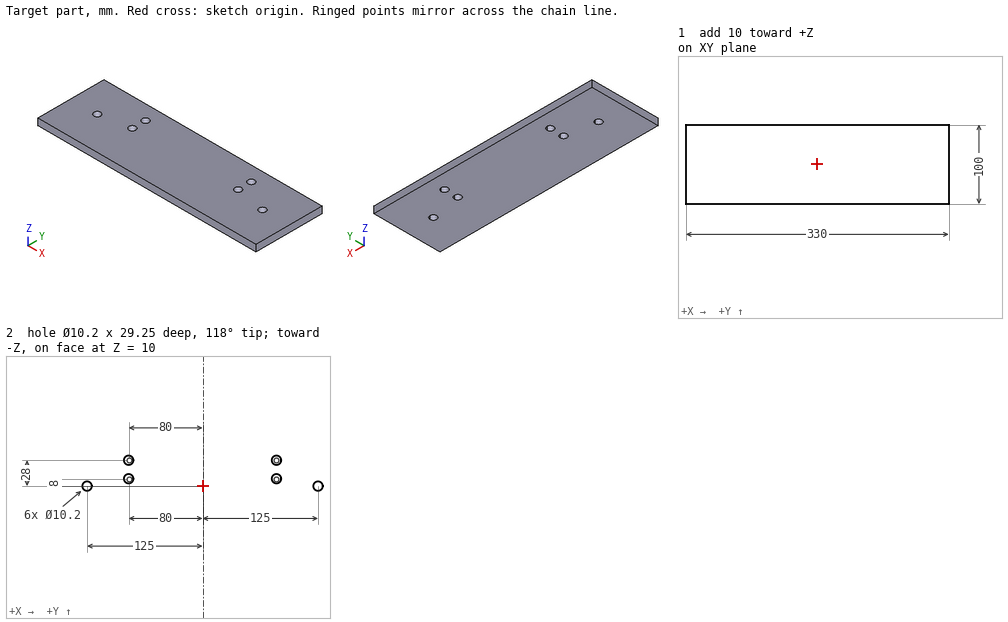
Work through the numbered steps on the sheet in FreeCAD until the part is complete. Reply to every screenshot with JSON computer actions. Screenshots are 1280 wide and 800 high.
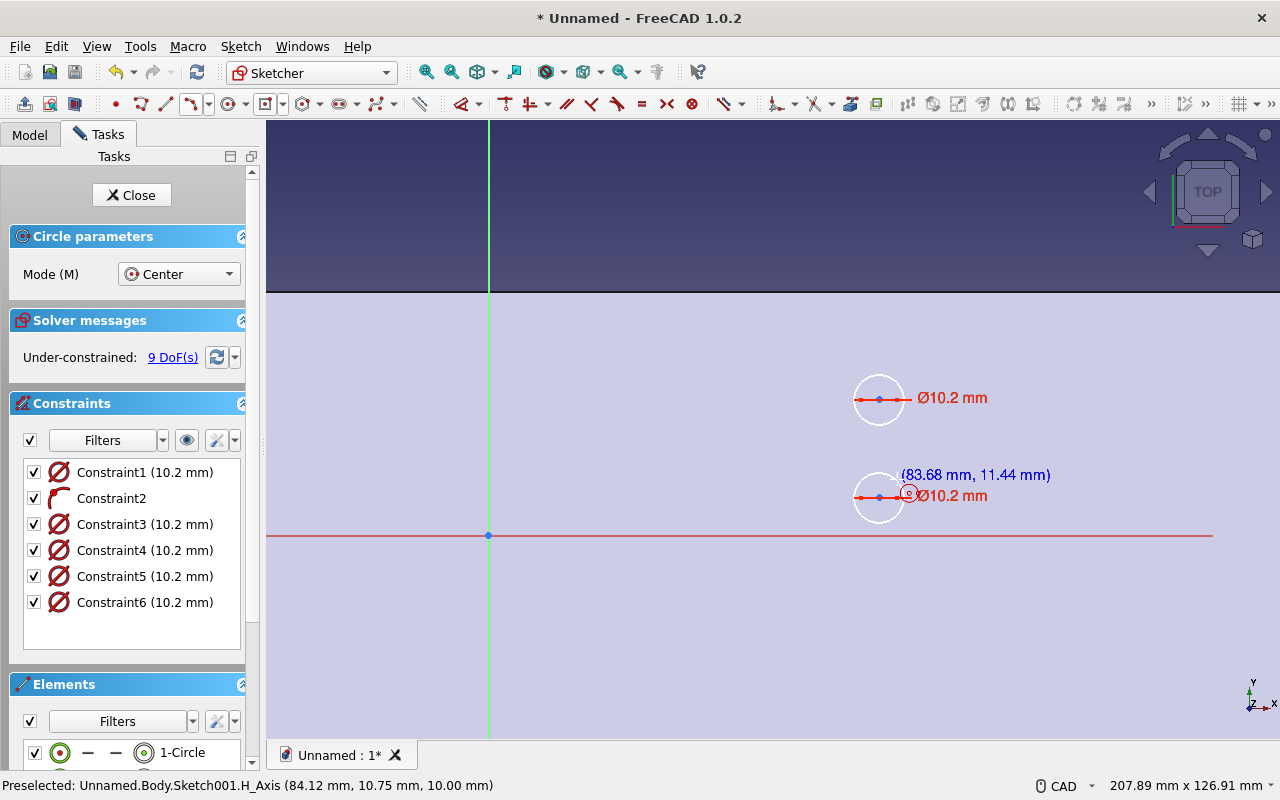
{"action": "left_click", "coordinate": [1099, 536]}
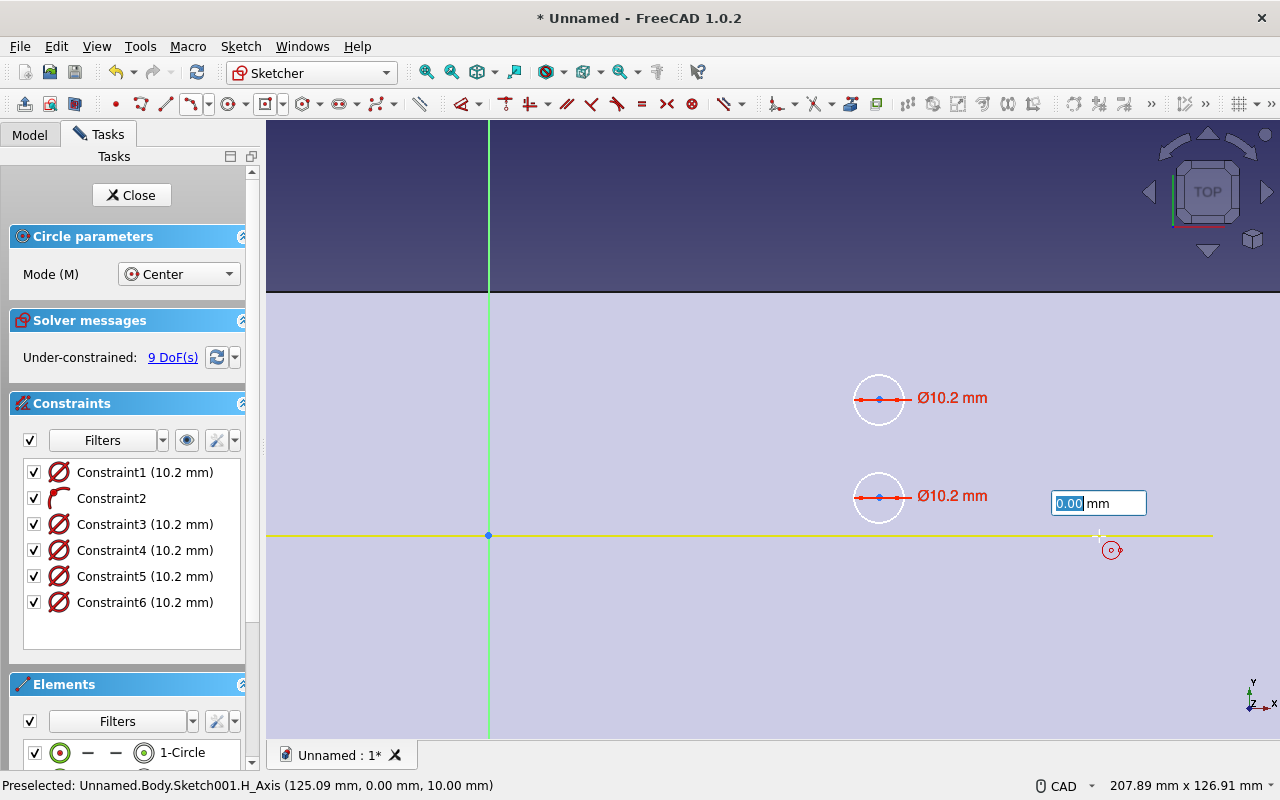
{"action": "scroll", "coordinate": [880, 398], "scroll_direction": "down", "scroll_amount": 4}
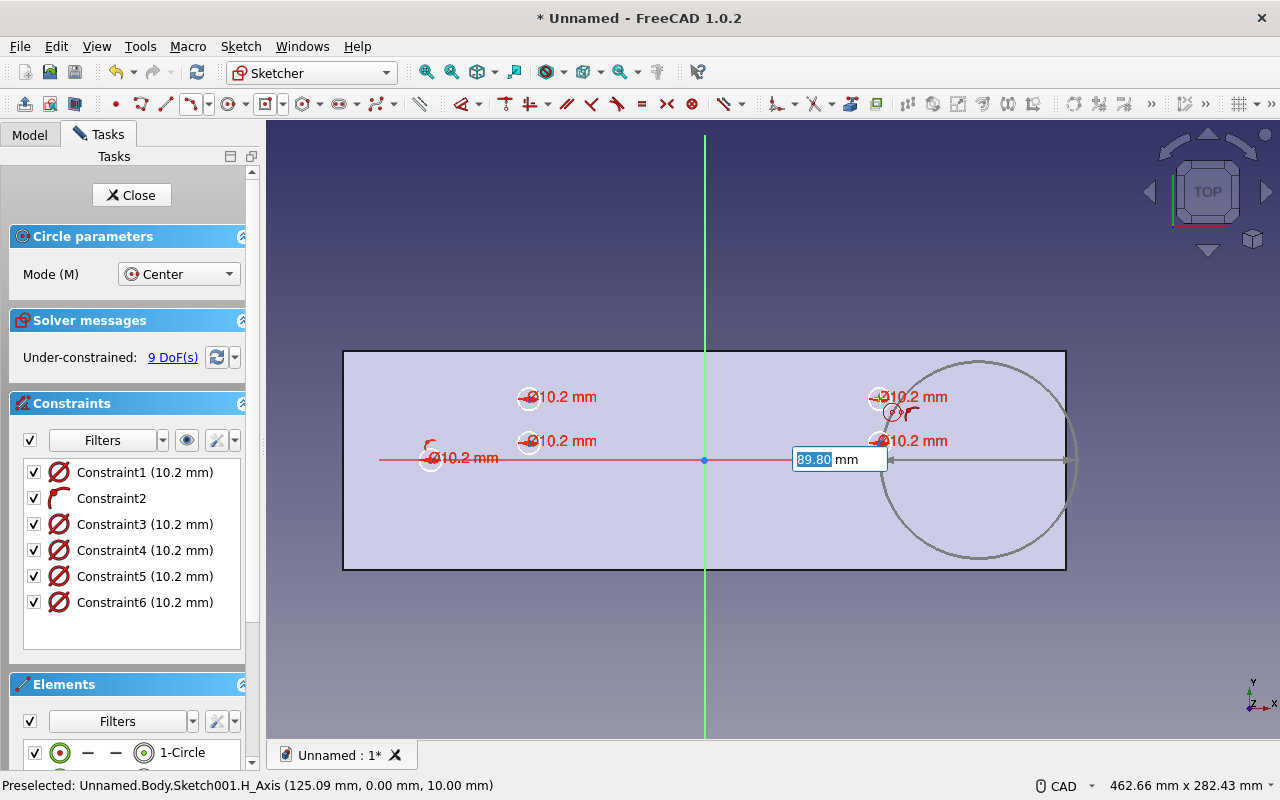
{"action": "scroll", "coordinate": [986, 452], "scroll_direction": "up", "scroll_amount": 4}
{"action": "mouse_move", "coordinate": [986, 452]}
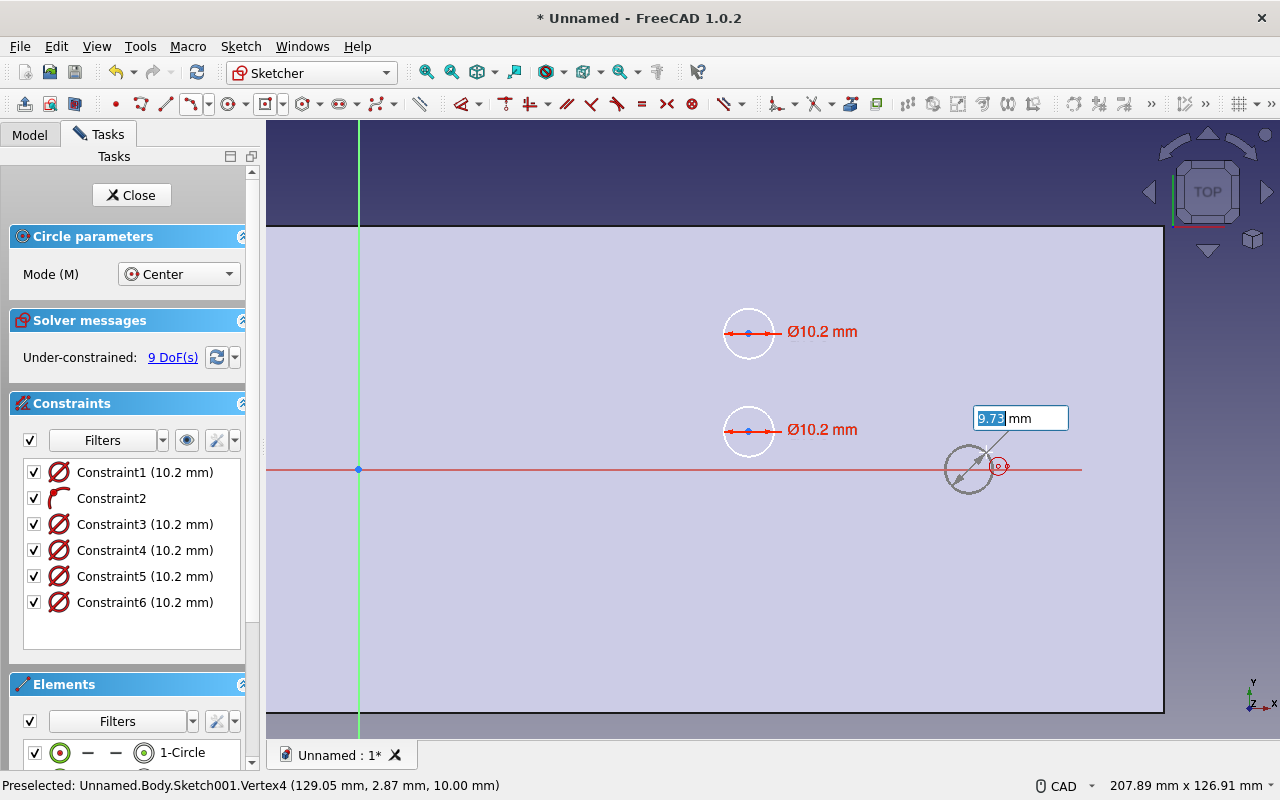
{"action": "type", "text": "10.2"}
{"action": "key", "text": "Return"}
{"action": "key", "text": "Escape"}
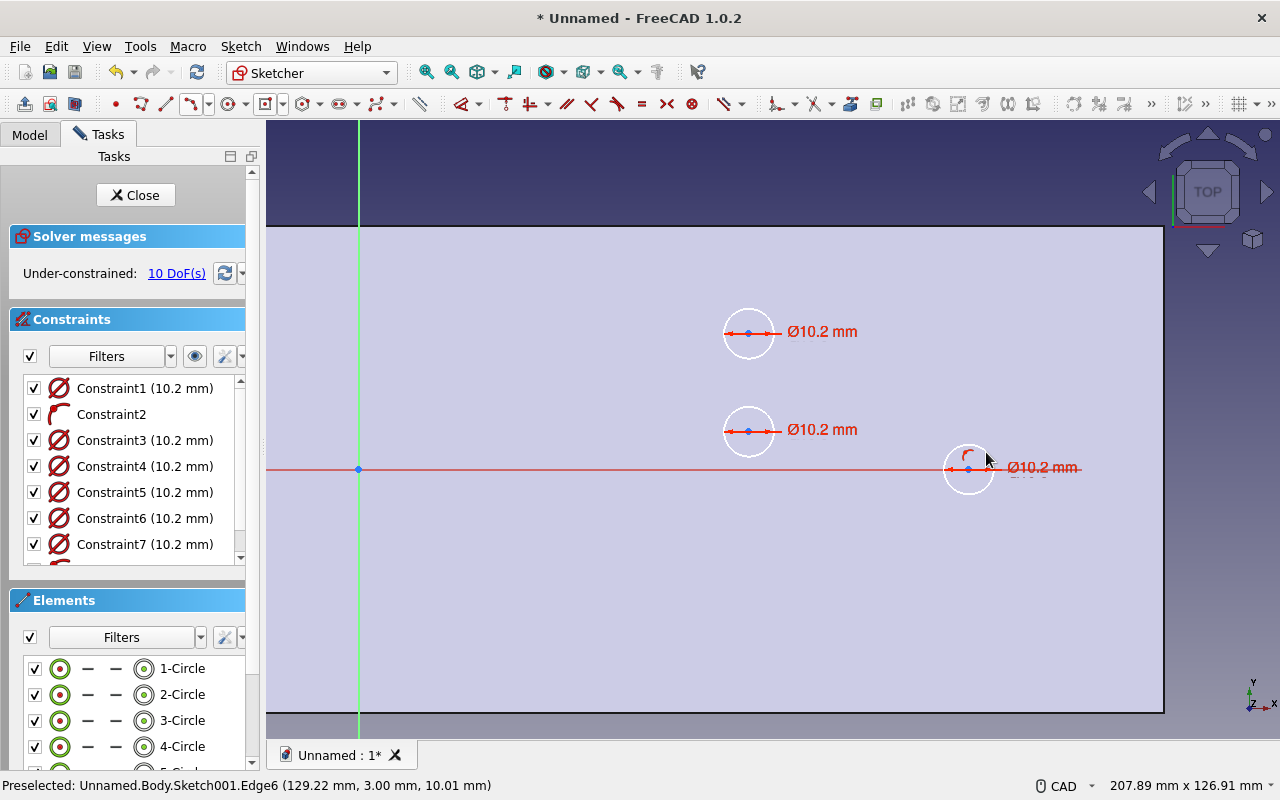
{"action": "scroll", "coordinate": [987, 453], "scroll_direction": "down", "scroll_amount": 4}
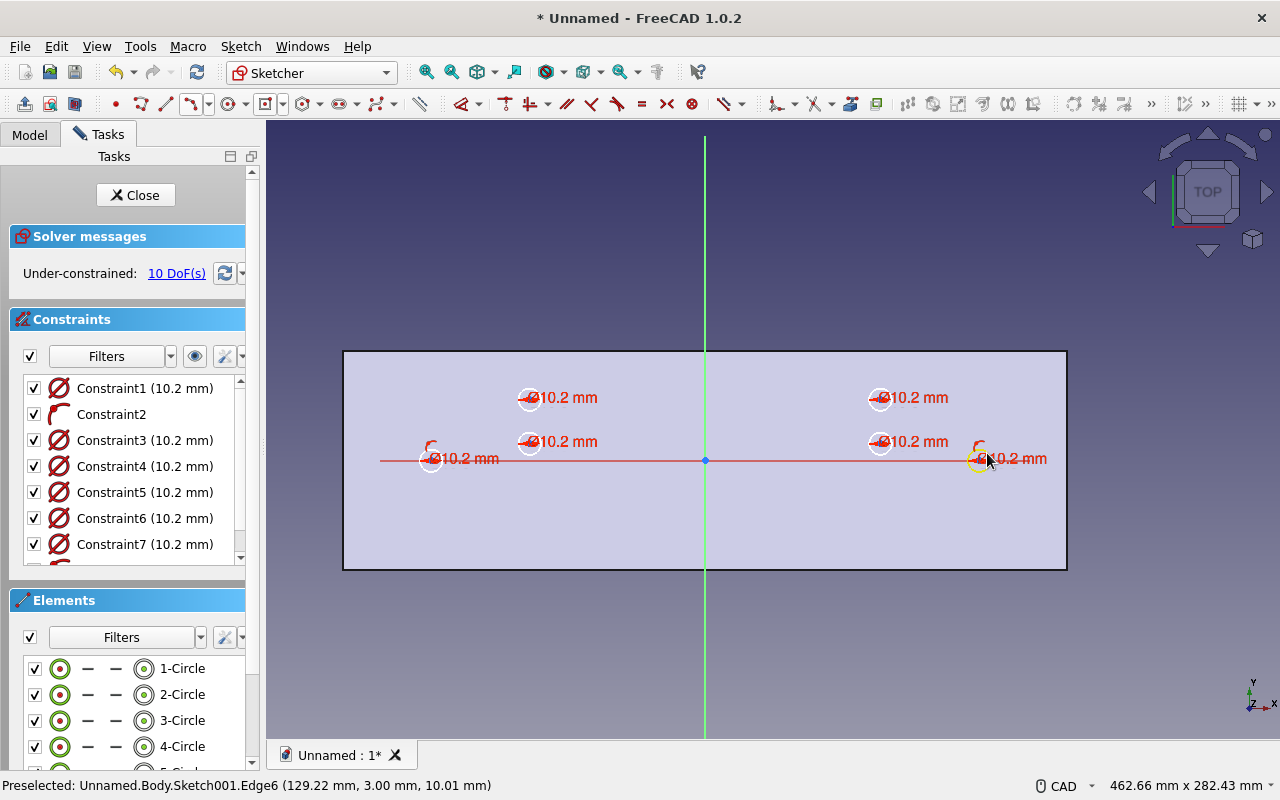
{"action": "left_click", "coordinate": [530, 400]}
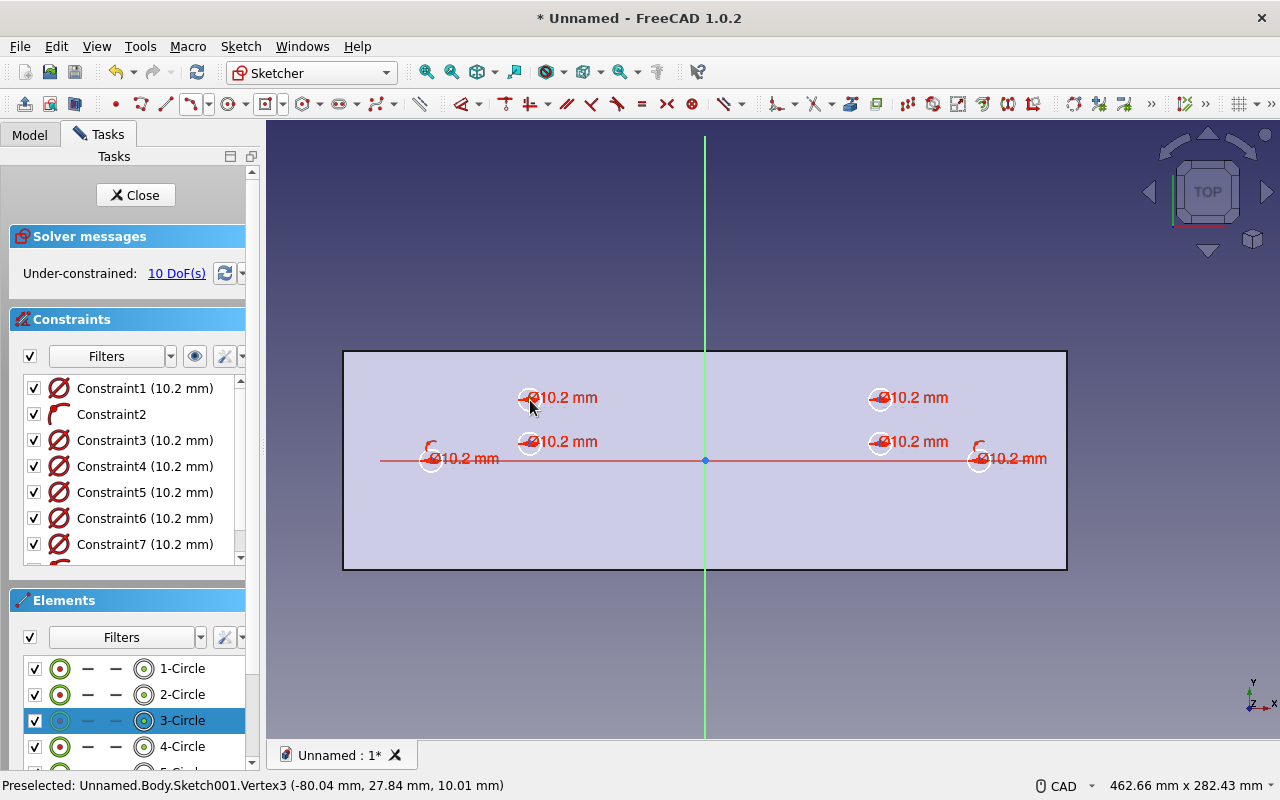
{"action": "left_click", "coordinate": [880, 400]}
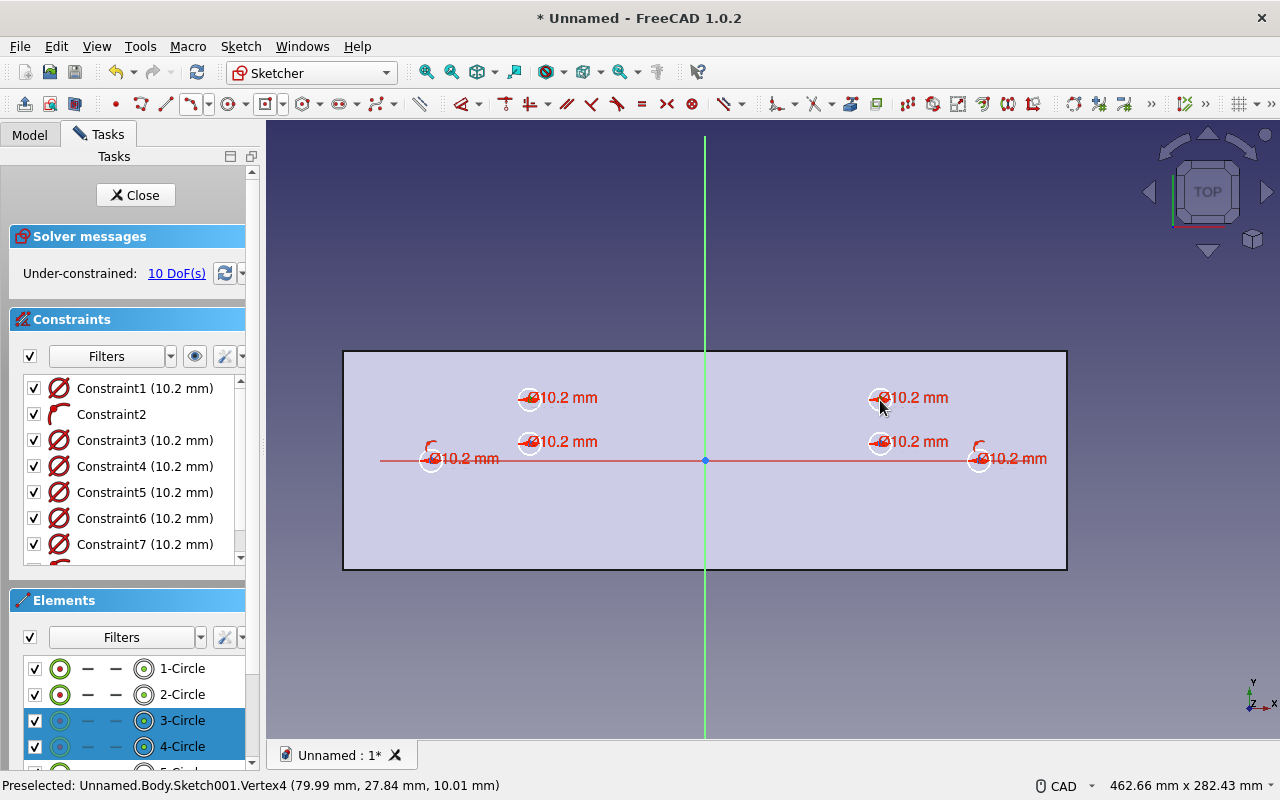
{"action": "left_click", "coordinate": [705, 671]}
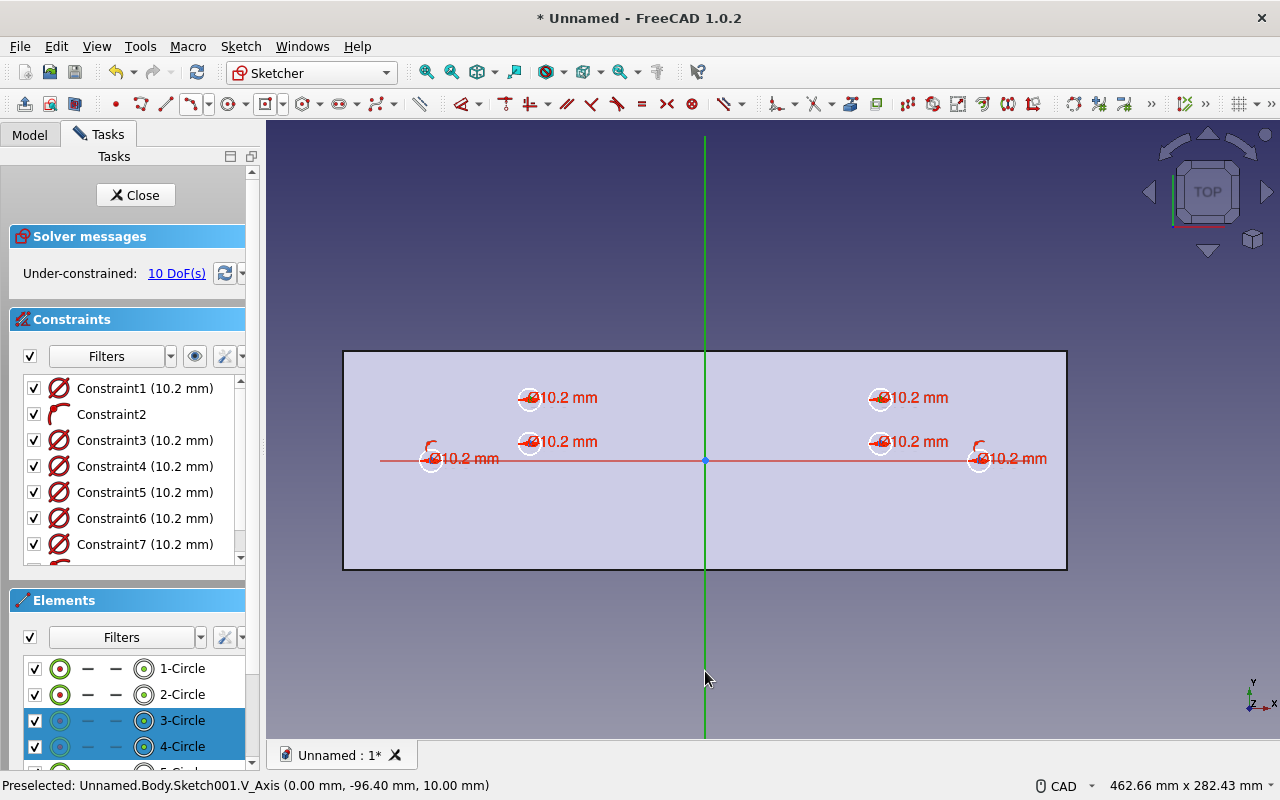
{"action": "left_click", "coordinate": [667, 104]}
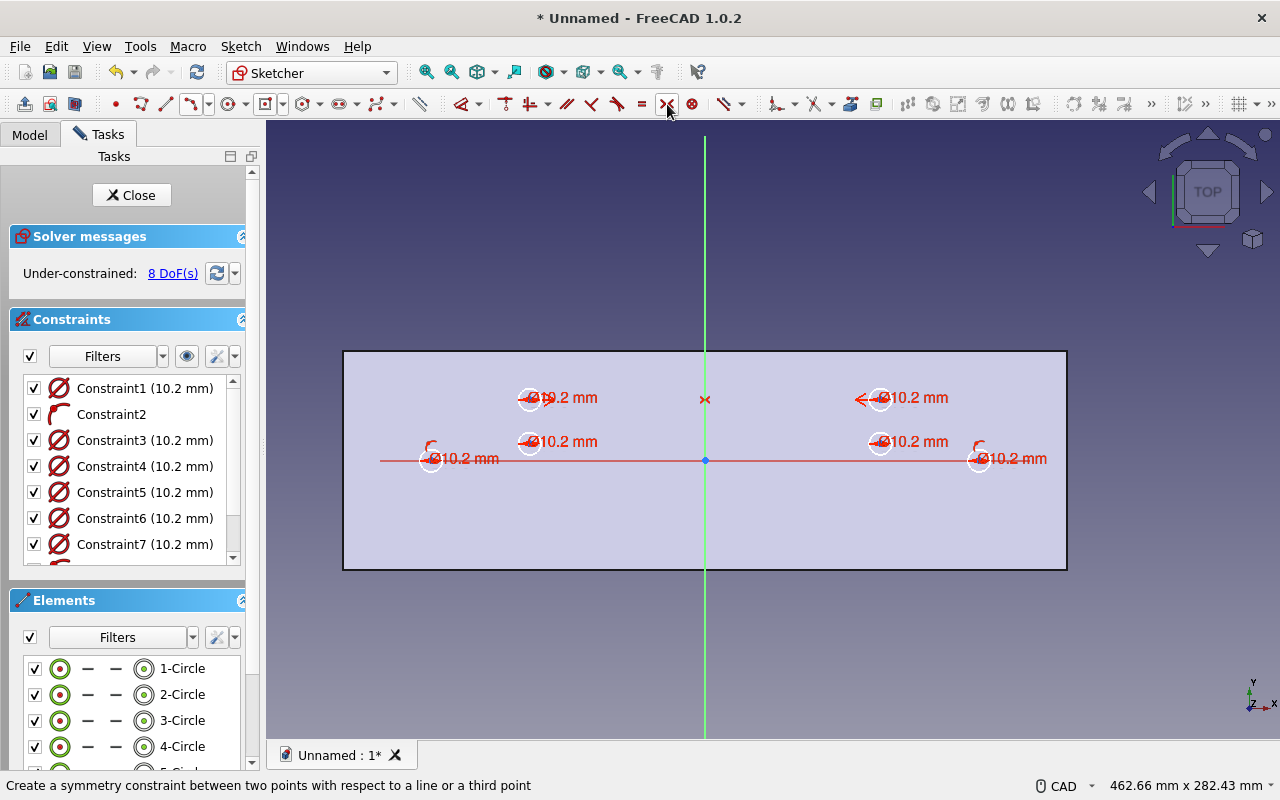
{"action": "left_click", "coordinate": [530, 444]}